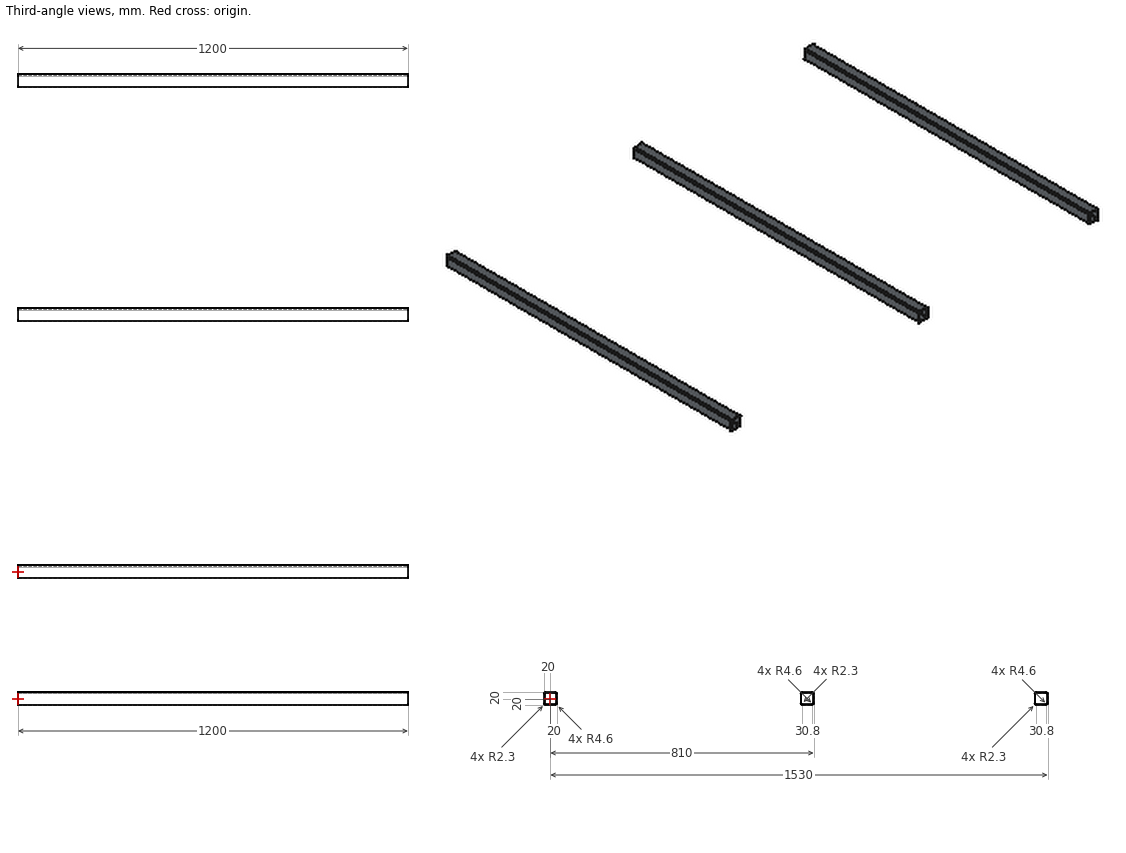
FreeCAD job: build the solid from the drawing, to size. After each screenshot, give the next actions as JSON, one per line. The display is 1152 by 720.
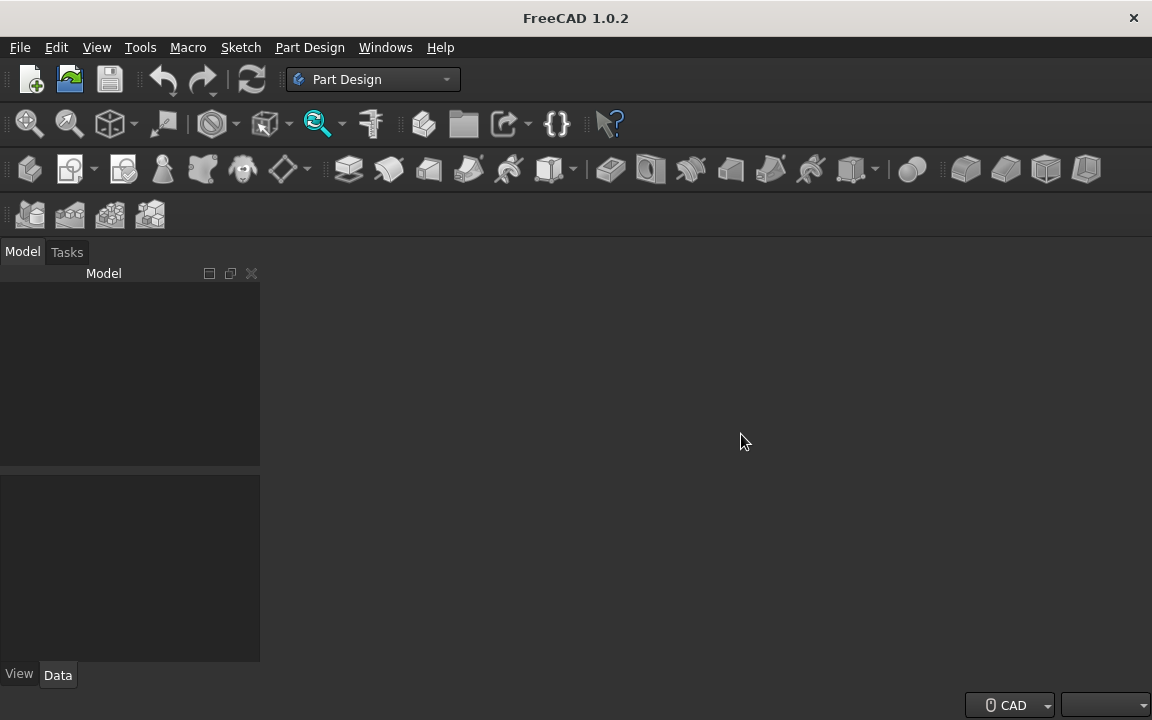
{"action": "left_click", "coordinate": [30, 80]}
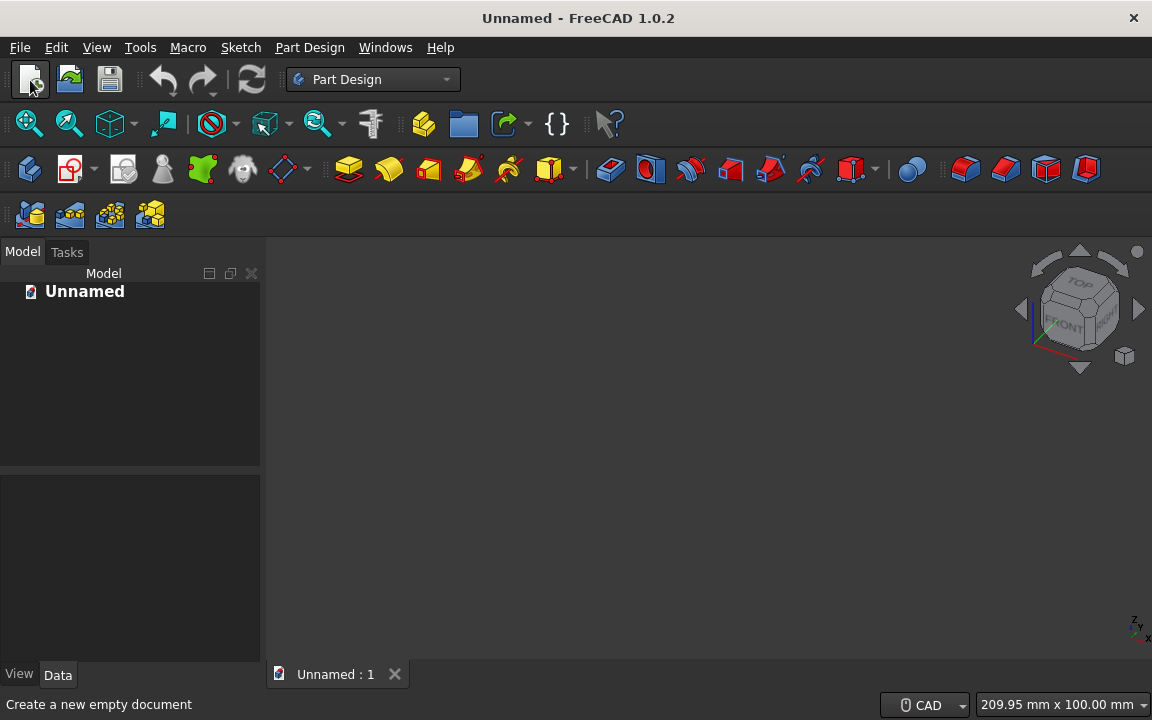
{"action": "left_click", "coordinate": [70, 170]}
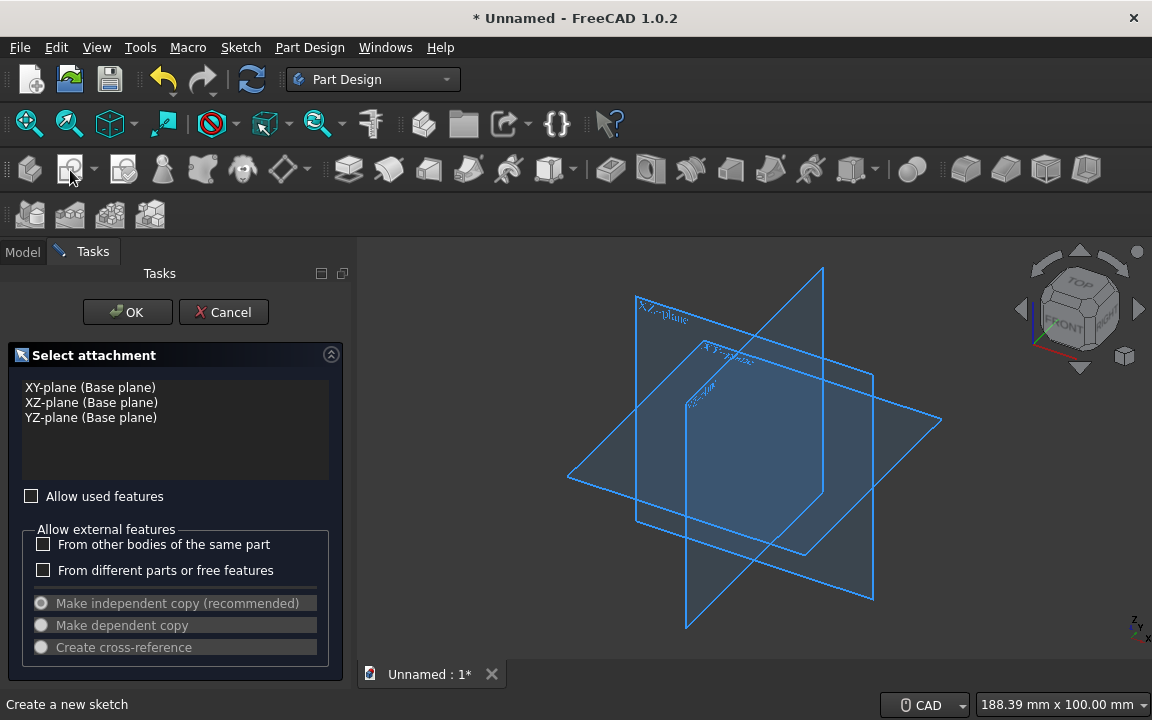
{"action": "left_click", "coordinate": [82, 418]}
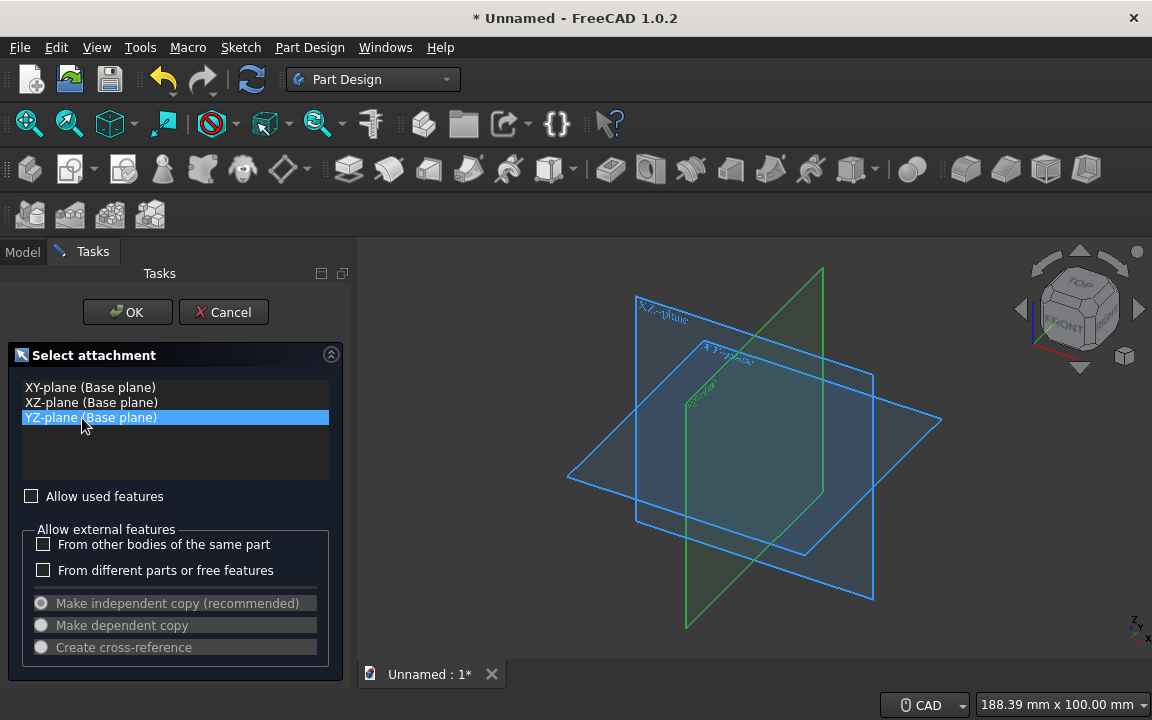
{"action": "left_click", "coordinate": [128, 312]}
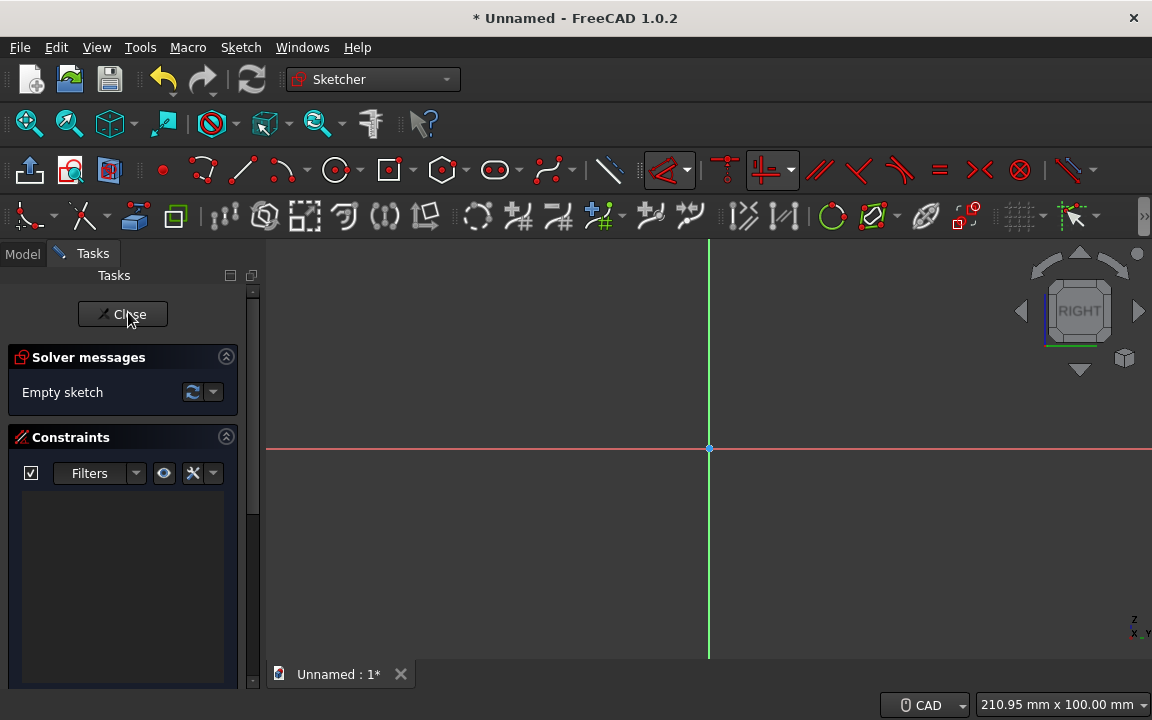
{"action": "scroll", "coordinate": [848, 449], "scroll_direction": "up", "scroll_amount": 2}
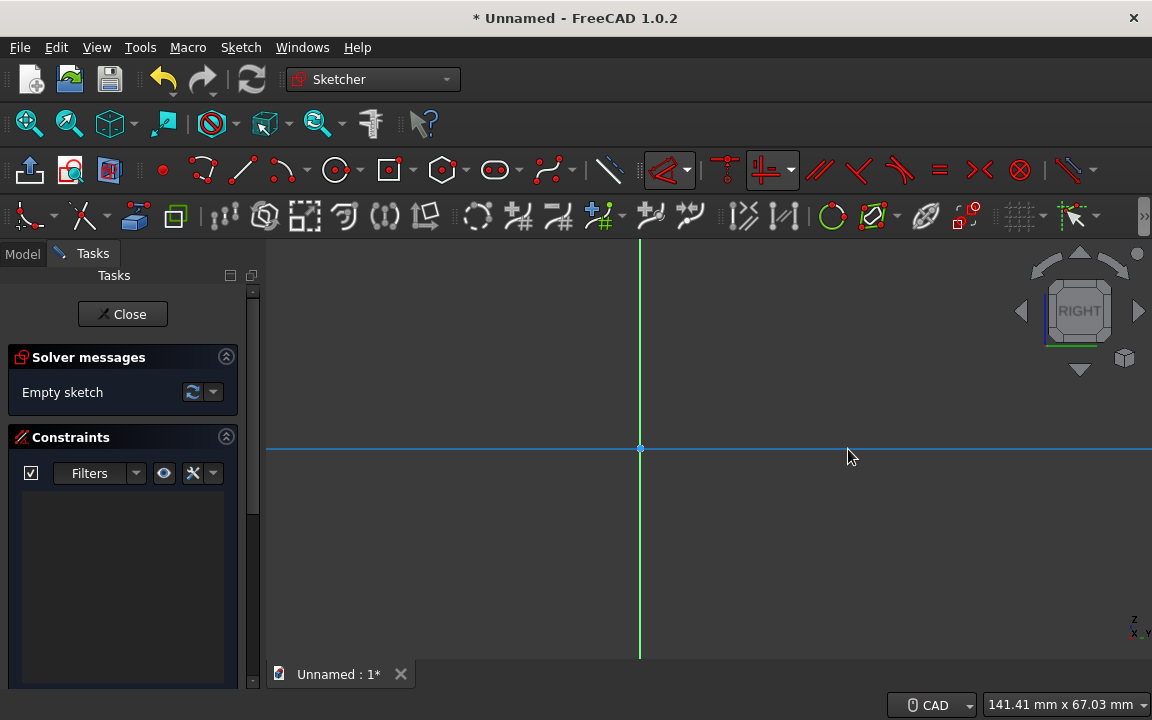
{"action": "key", "text": "g l"}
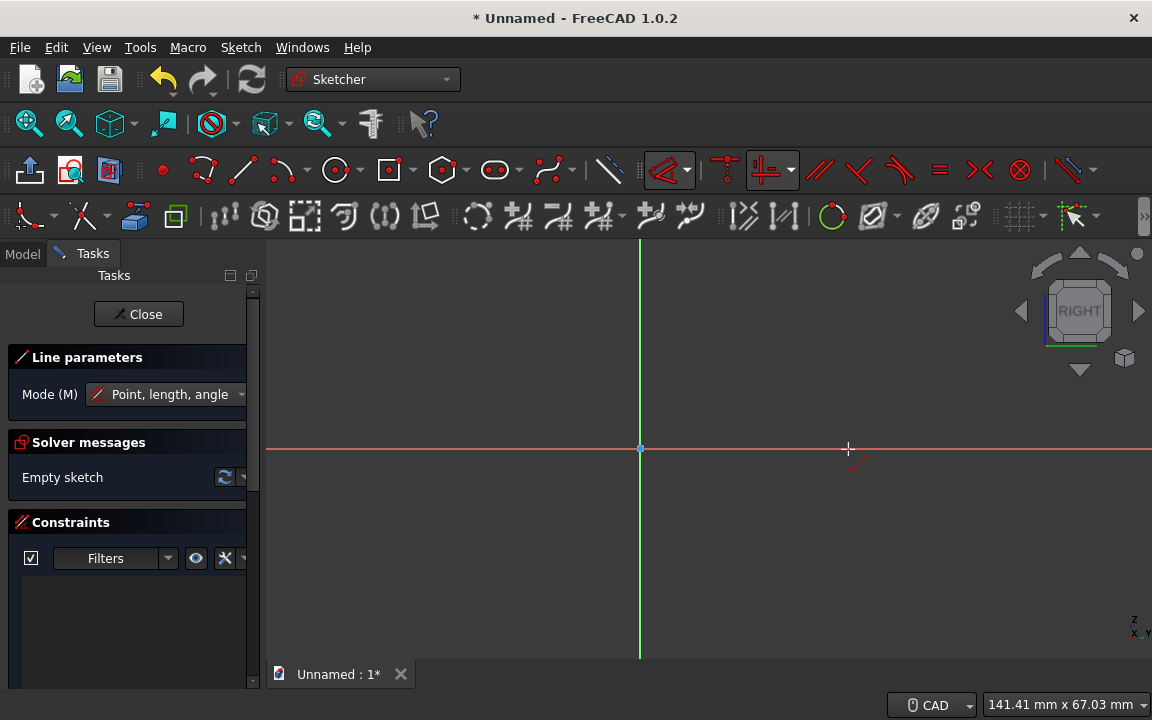
{"action": "left_click", "coordinate": [544, 574]}
{"action": "left_click", "coordinate": [737, 574]}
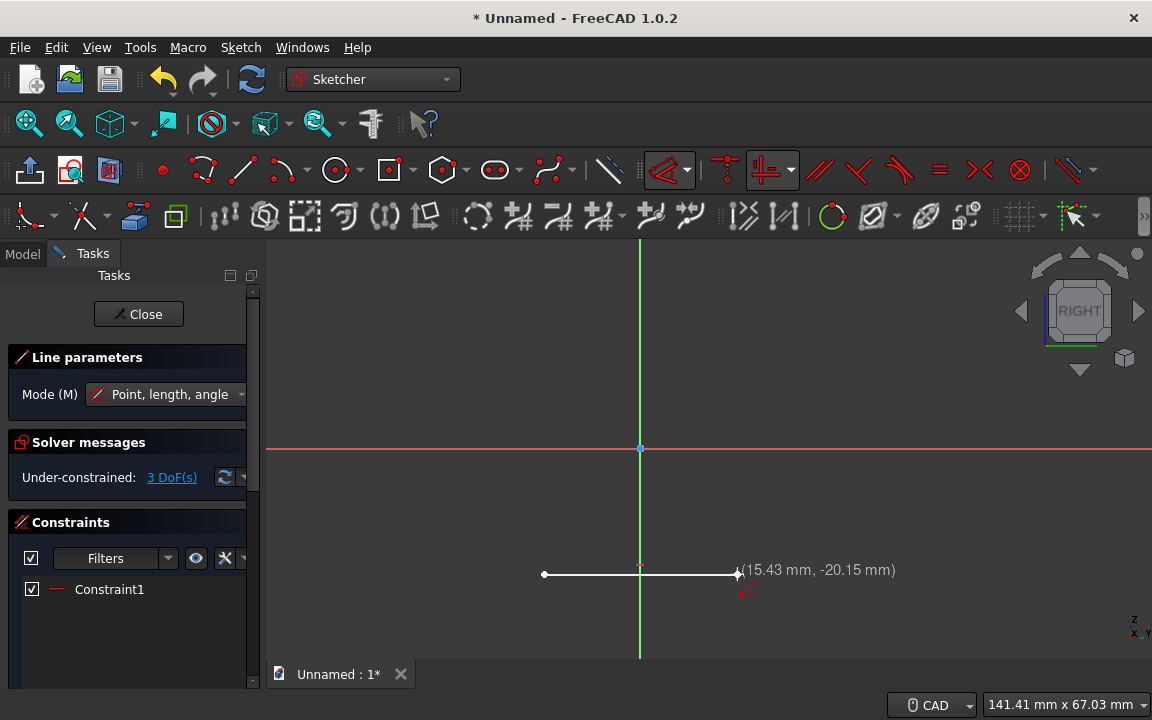
{"action": "left_click", "coordinate": [766, 545]}
{"action": "left_click", "coordinate": [766, 352]}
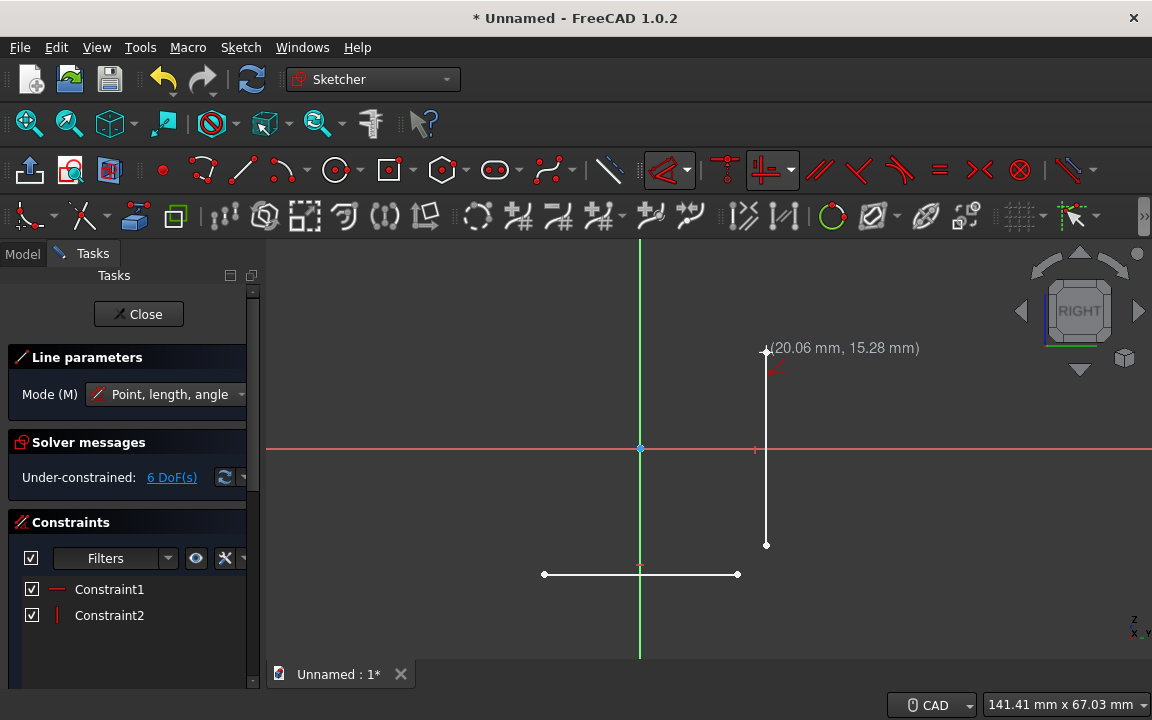
{"action": "left_click", "coordinate": [737, 323]}
{"action": "left_click", "coordinate": [544, 323]}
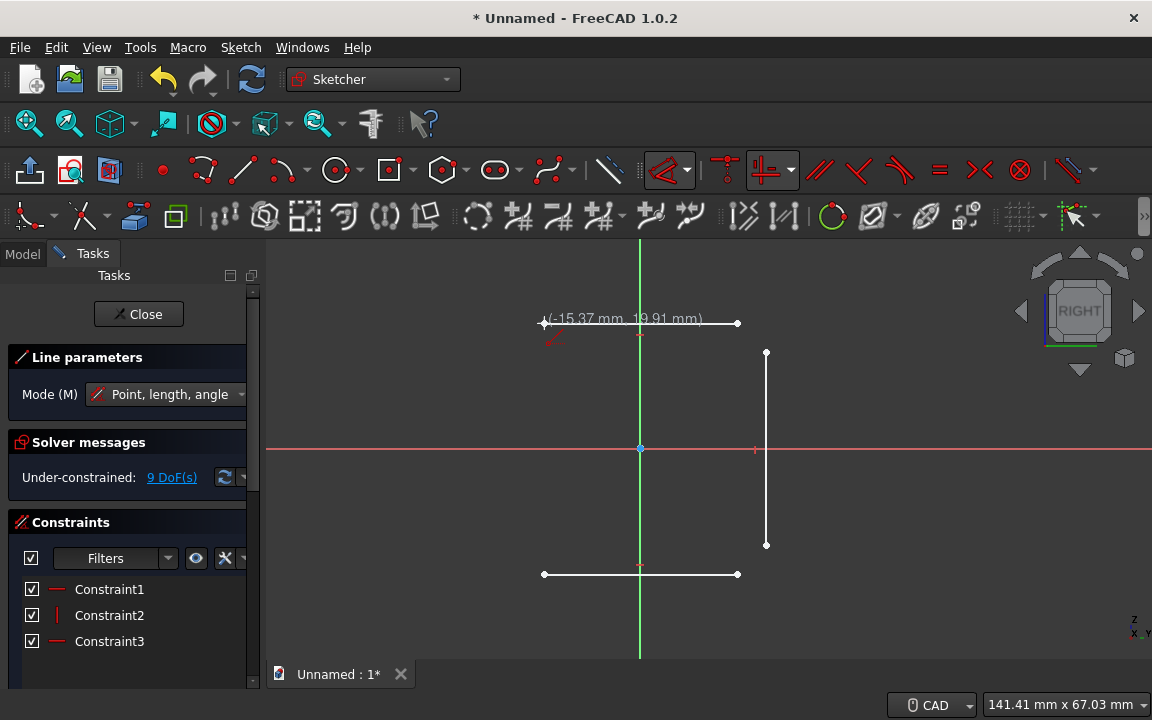
{"action": "left_click", "coordinate": [515, 352]}
{"action": "left_click", "coordinate": [515, 545]}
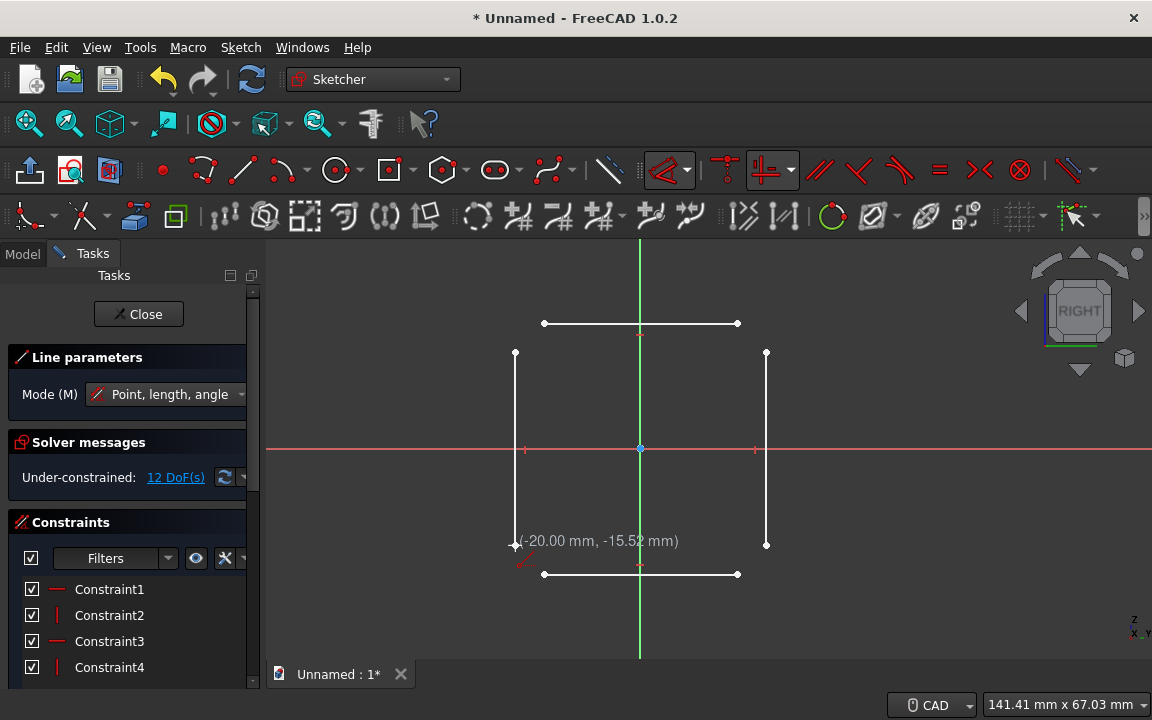
{"action": "key", "text": "g 3 a"}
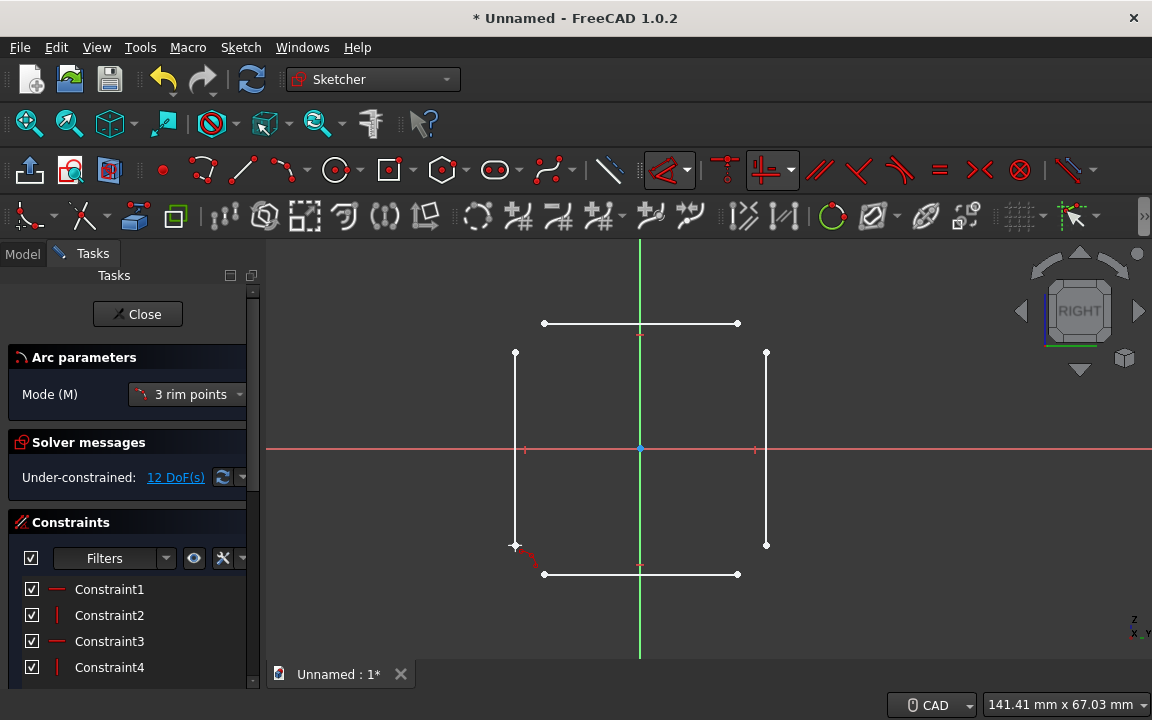
{"action": "left_click", "coordinate": [737, 575]}
{"action": "left_click", "coordinate": [766, 546]}